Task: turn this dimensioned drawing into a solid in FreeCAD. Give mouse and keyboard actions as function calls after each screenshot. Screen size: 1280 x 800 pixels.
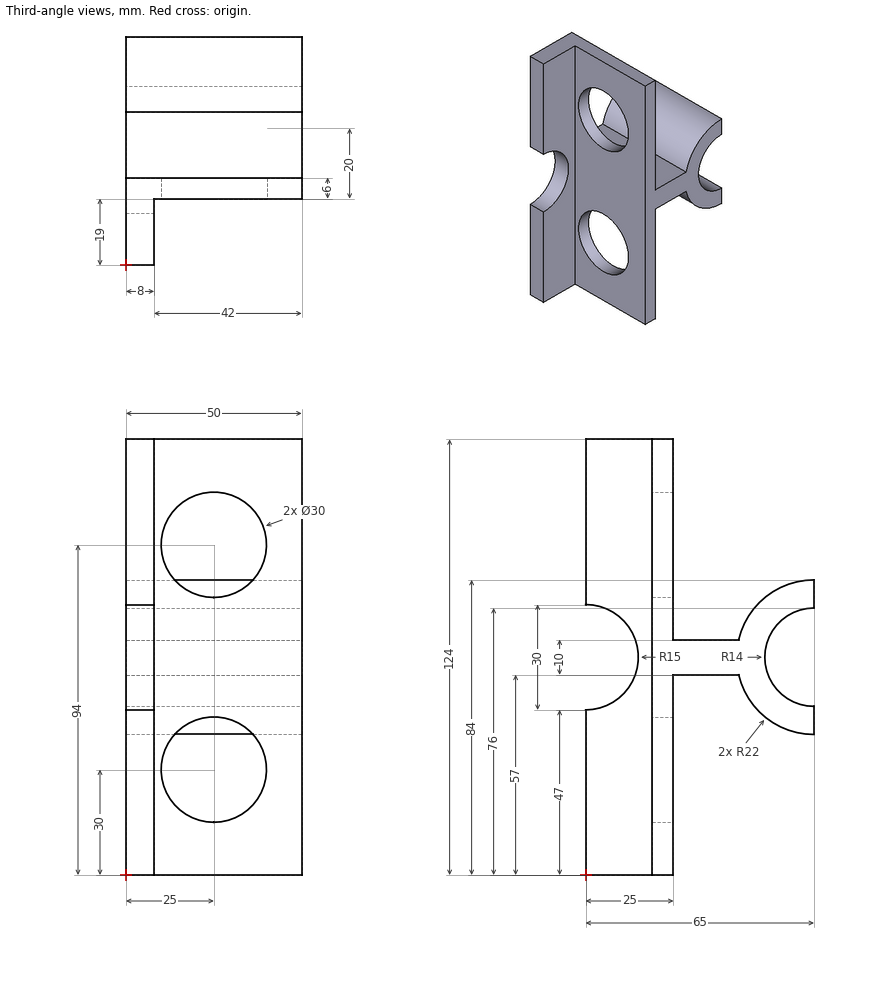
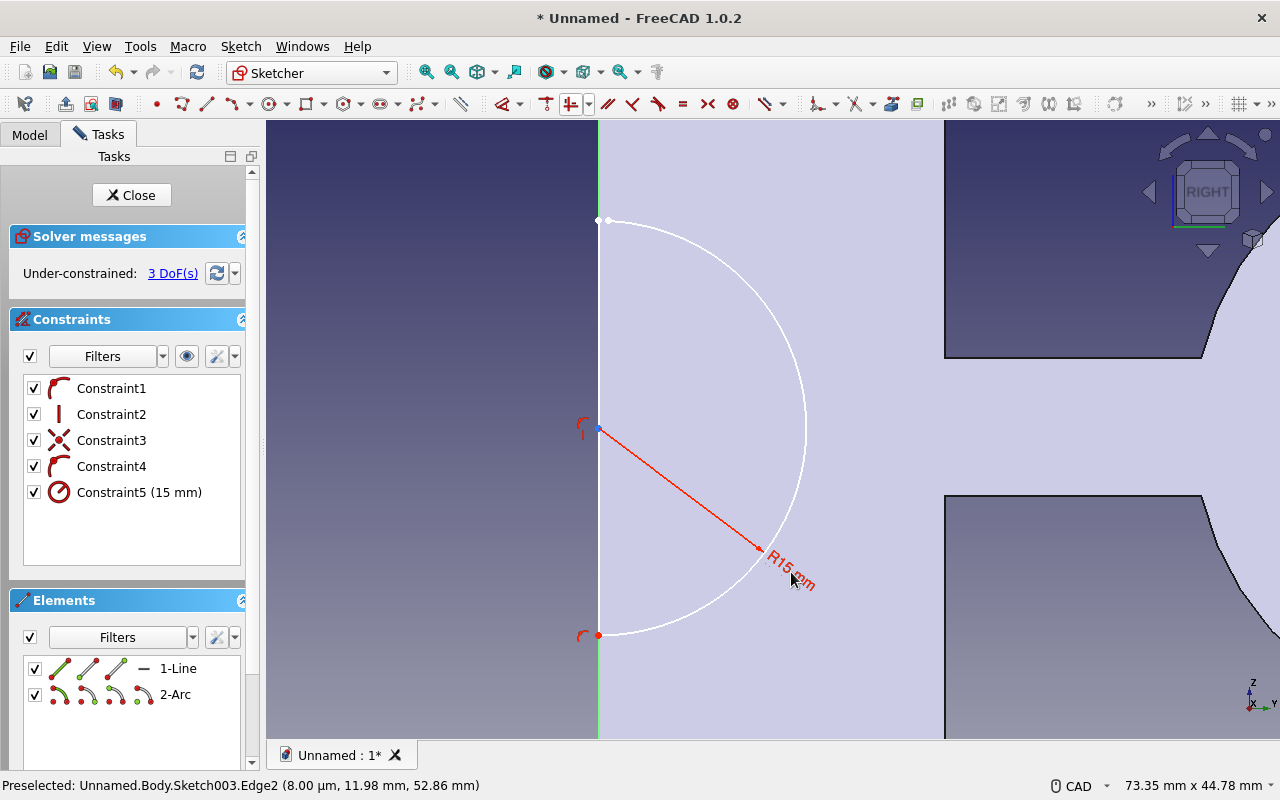
click(608, 221)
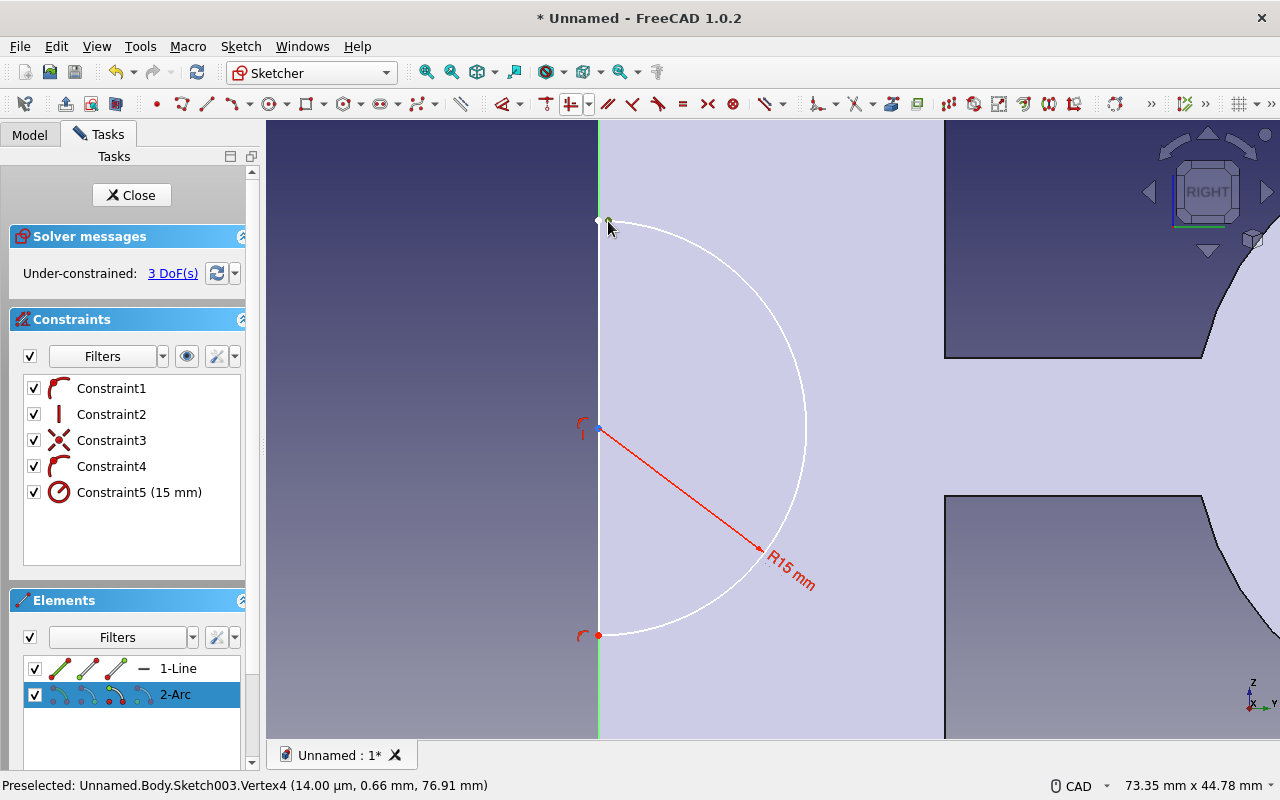
click(599, 671)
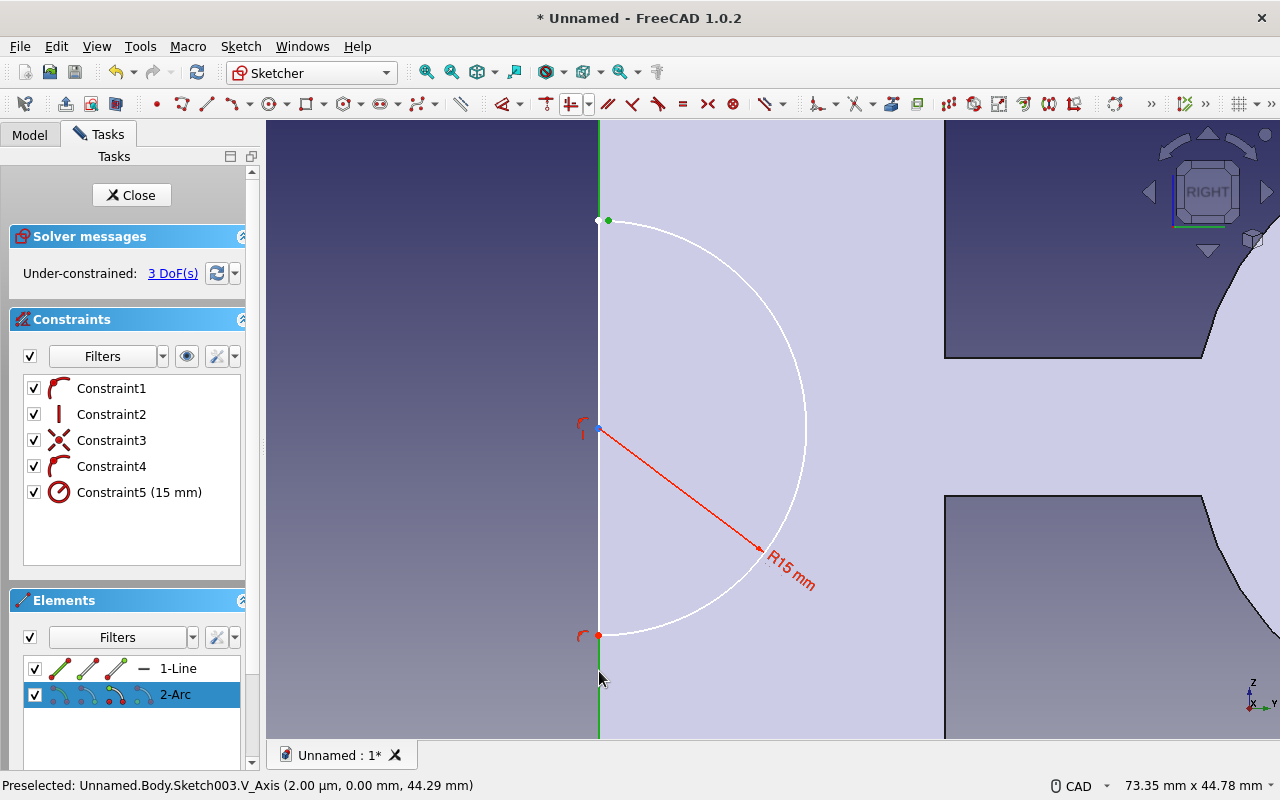
key(c)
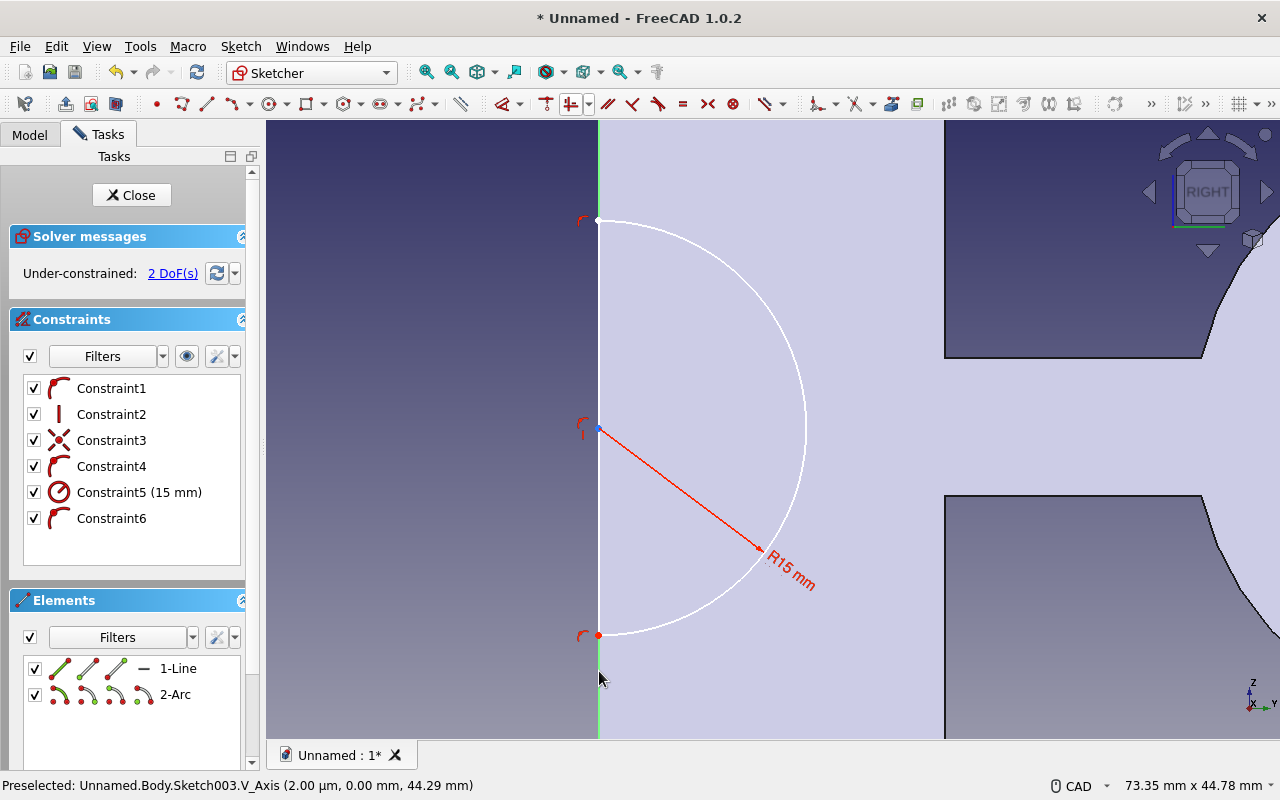
click(502, 104)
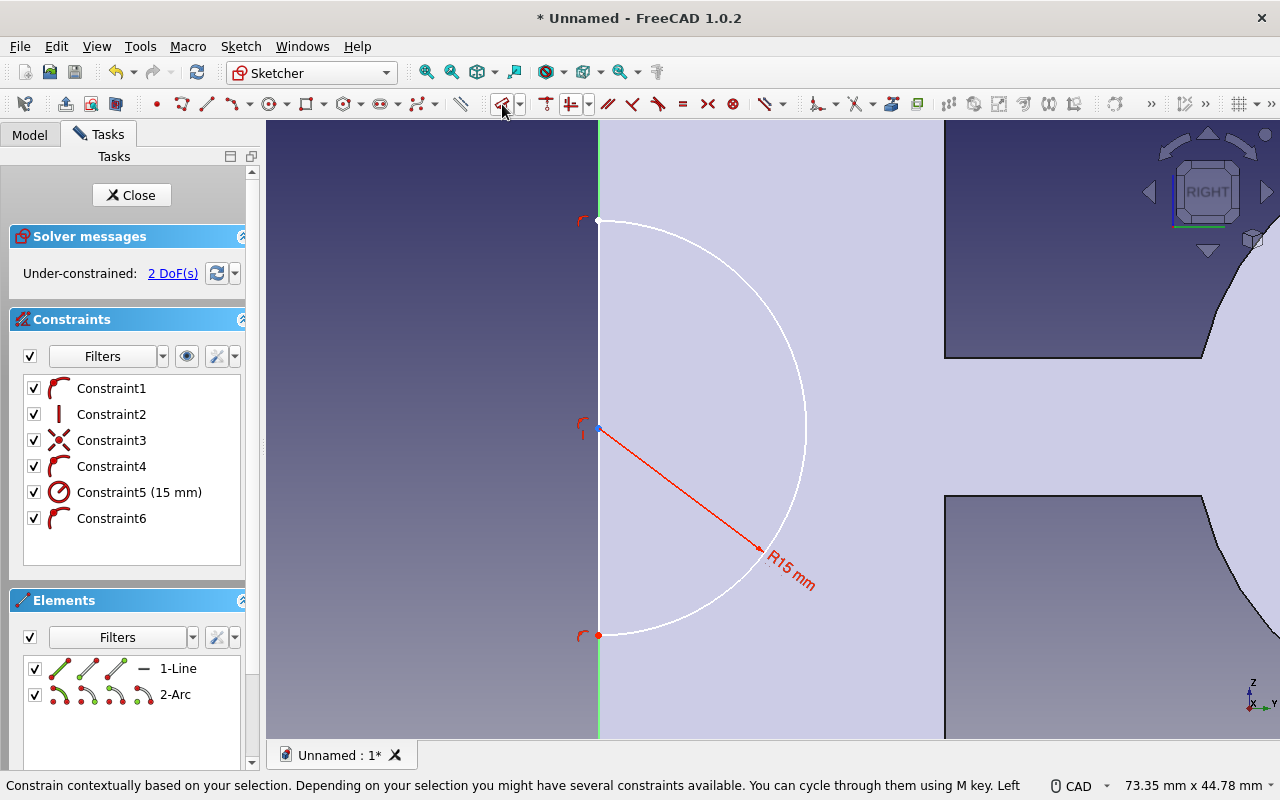
click(599, 511)
click(565, 428)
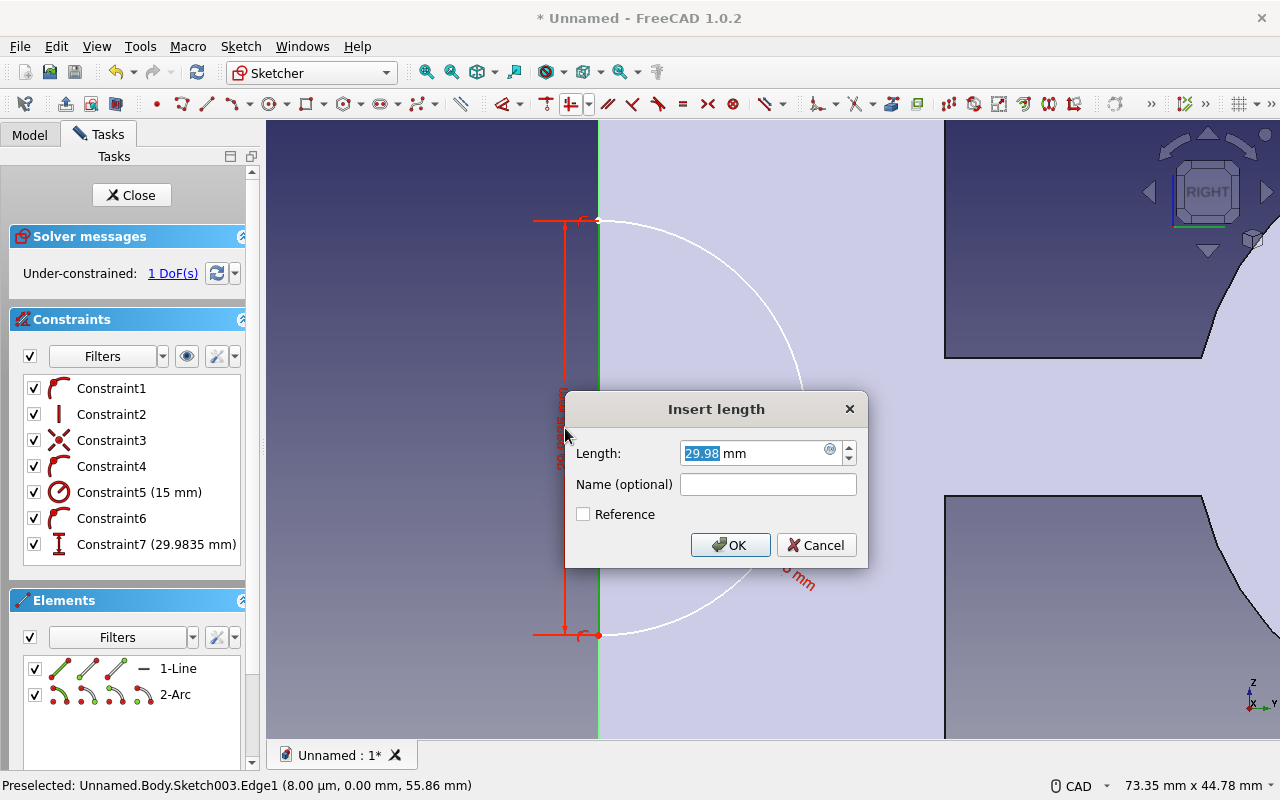
text(30)
key(Return)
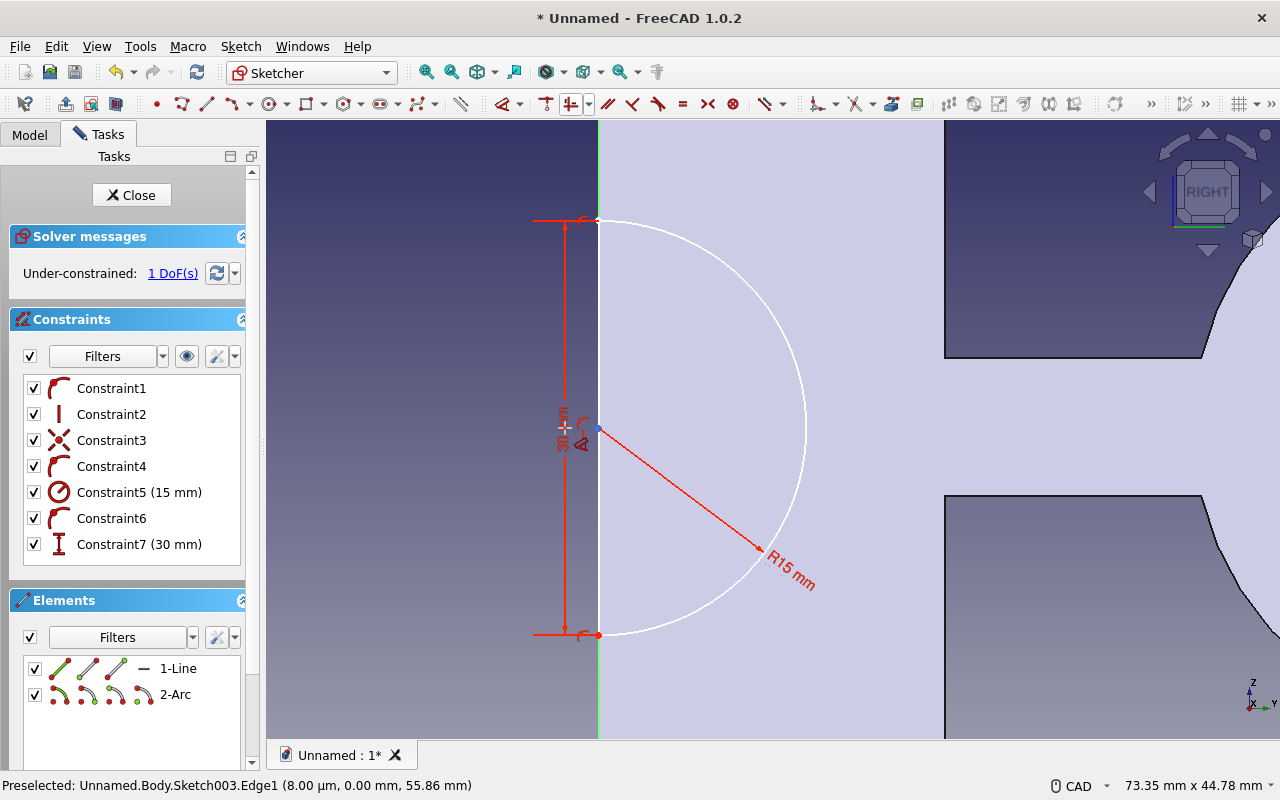
click(599, 635)
click(565, 673)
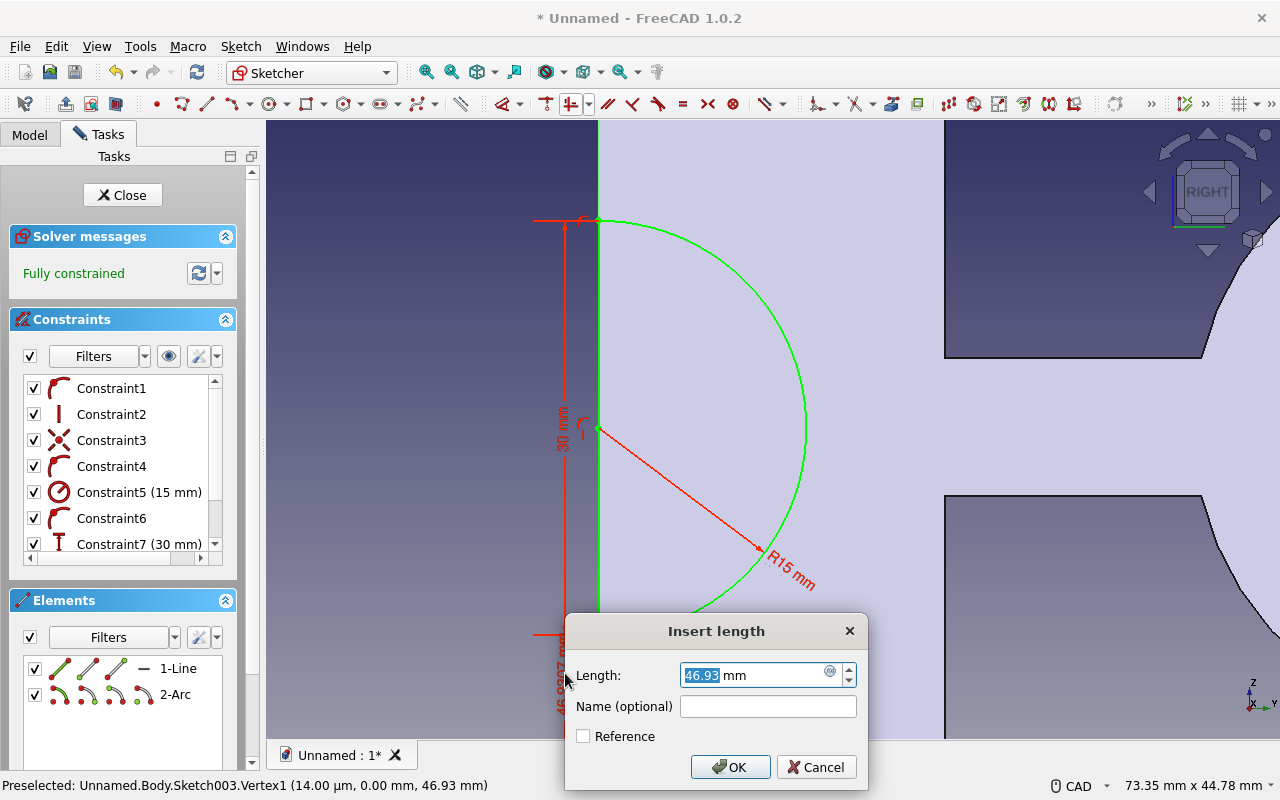
text(47)
key(Return)
key(Escape)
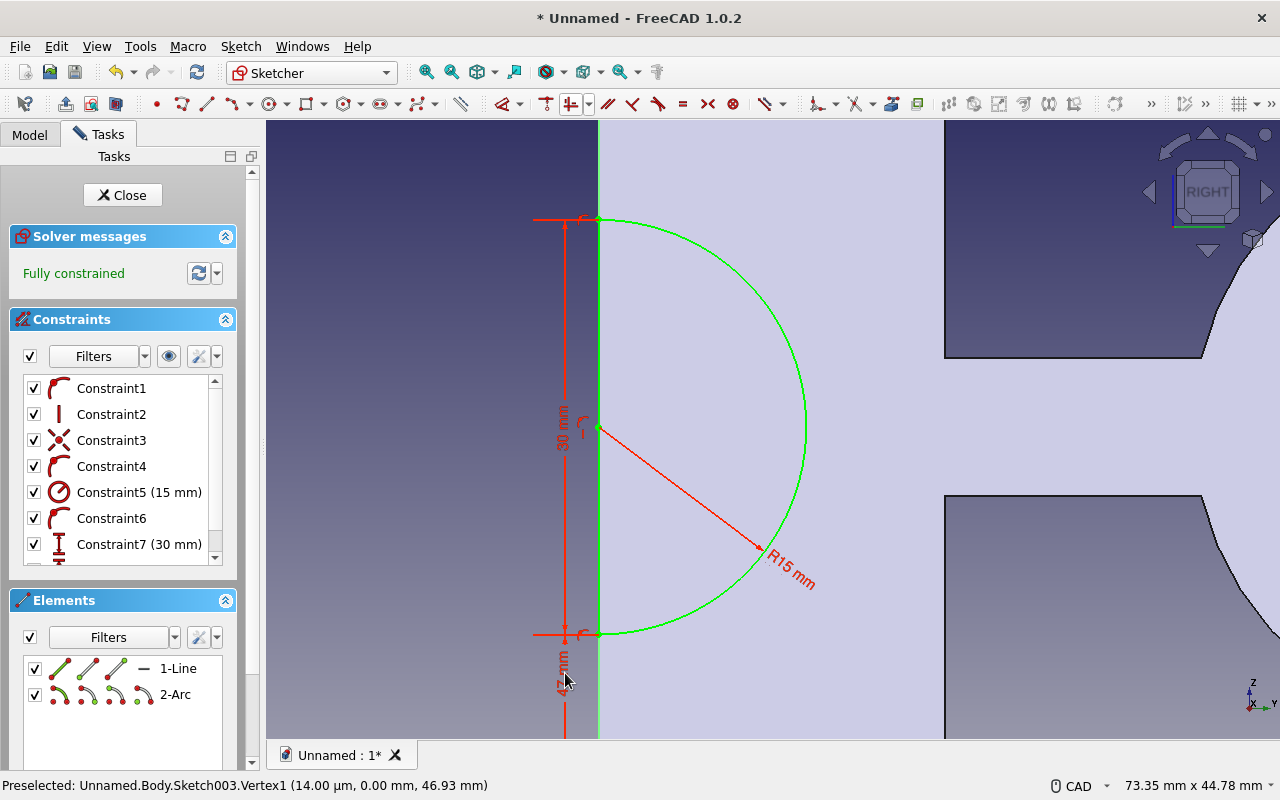
click(123, 195)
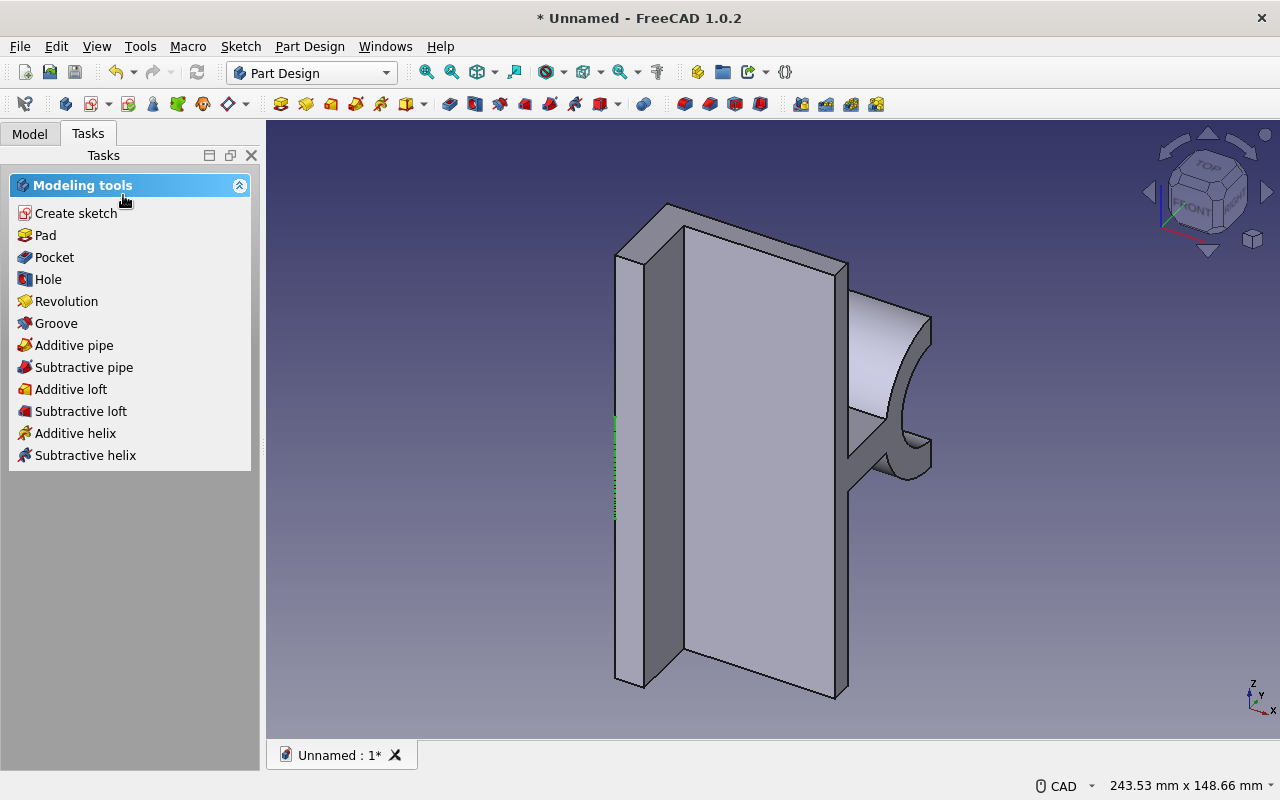
click(450, 104)